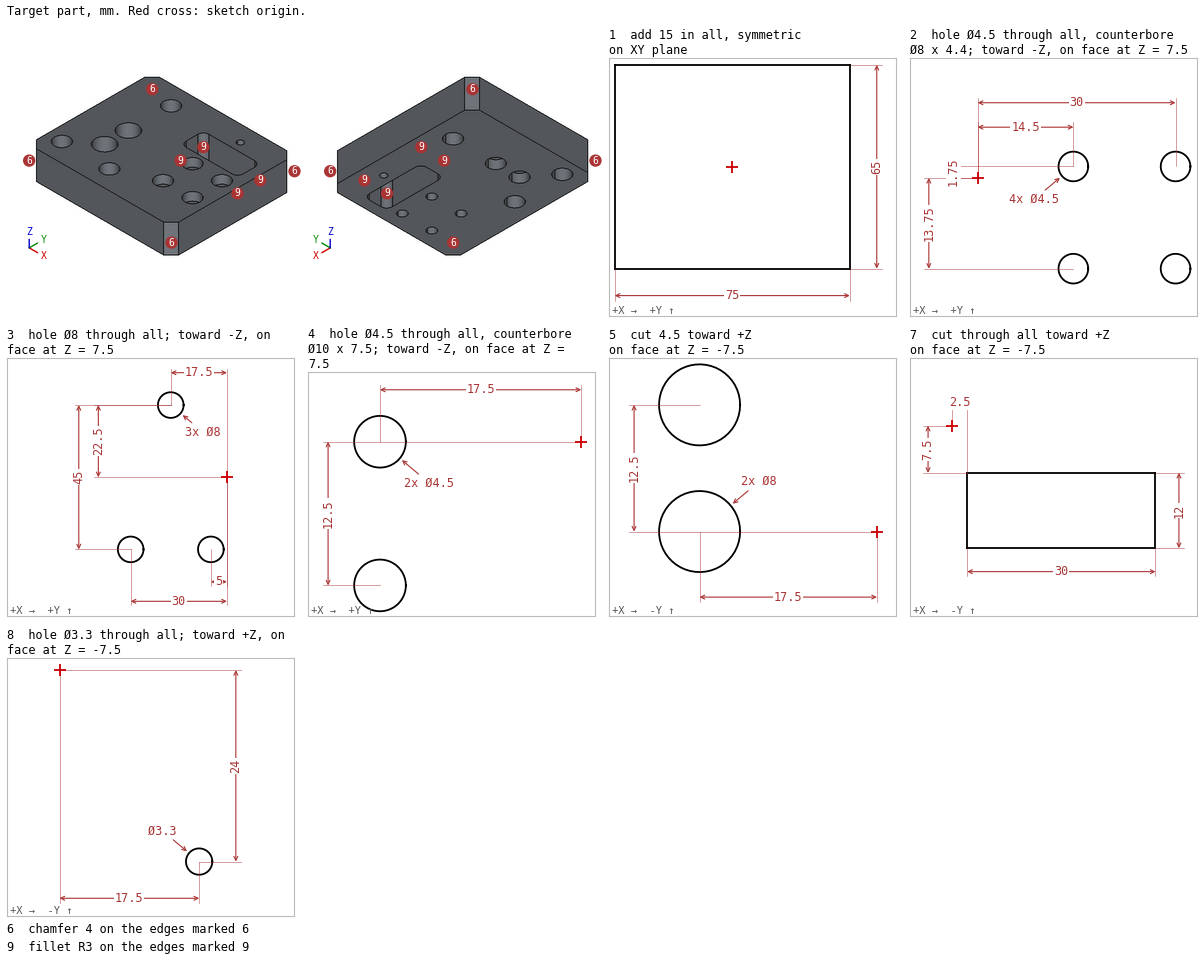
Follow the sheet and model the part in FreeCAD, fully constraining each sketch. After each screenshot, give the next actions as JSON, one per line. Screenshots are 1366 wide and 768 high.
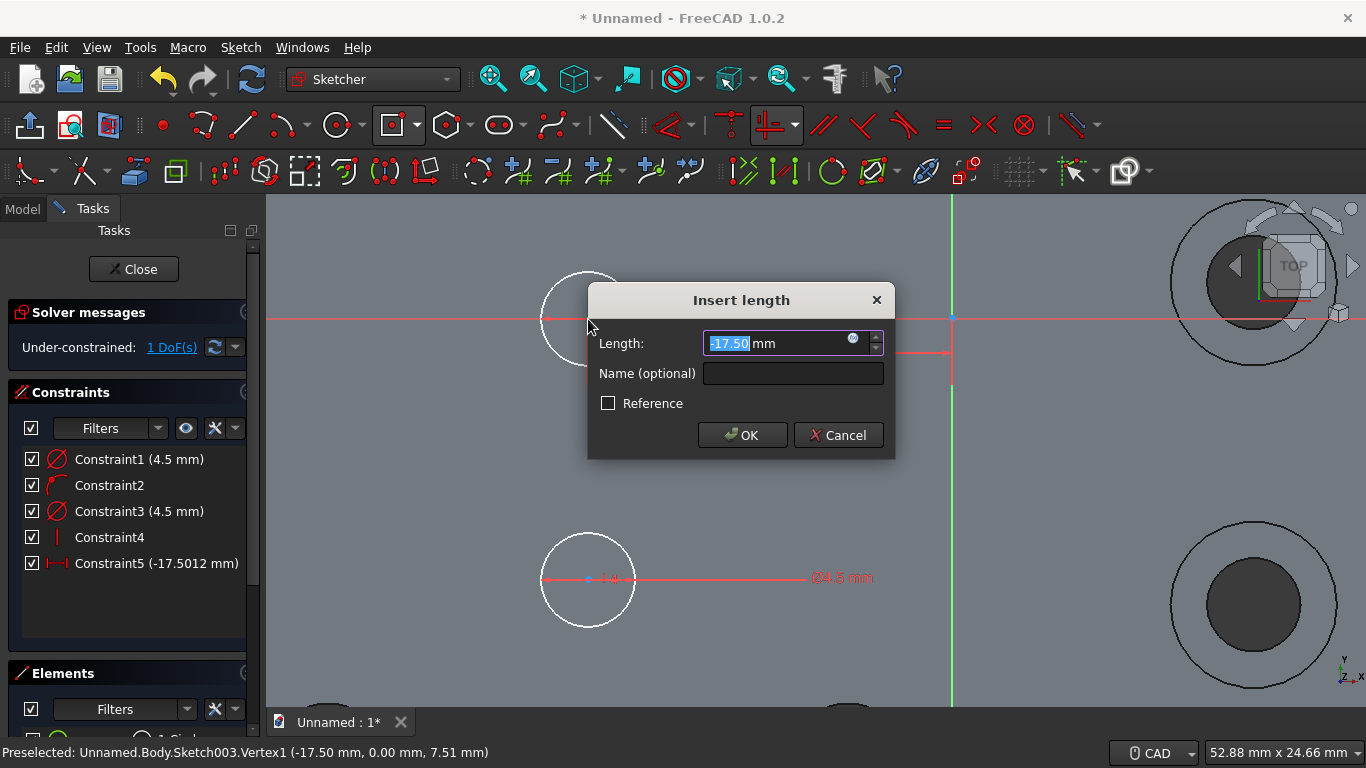
{"action": "type", "text": "-17.5"}
{"action": "key", "text": "Return"}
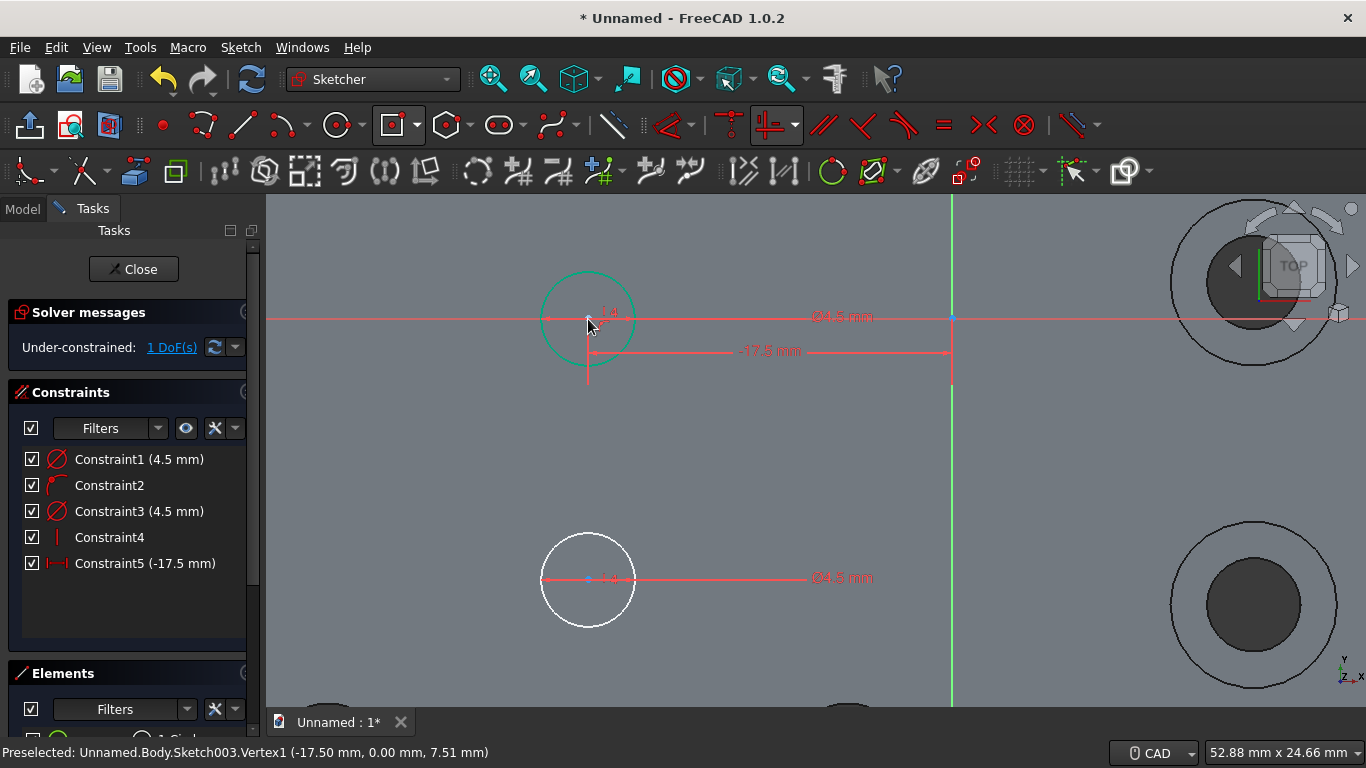
{"action": "left_click", "coordinate": [588, 580]}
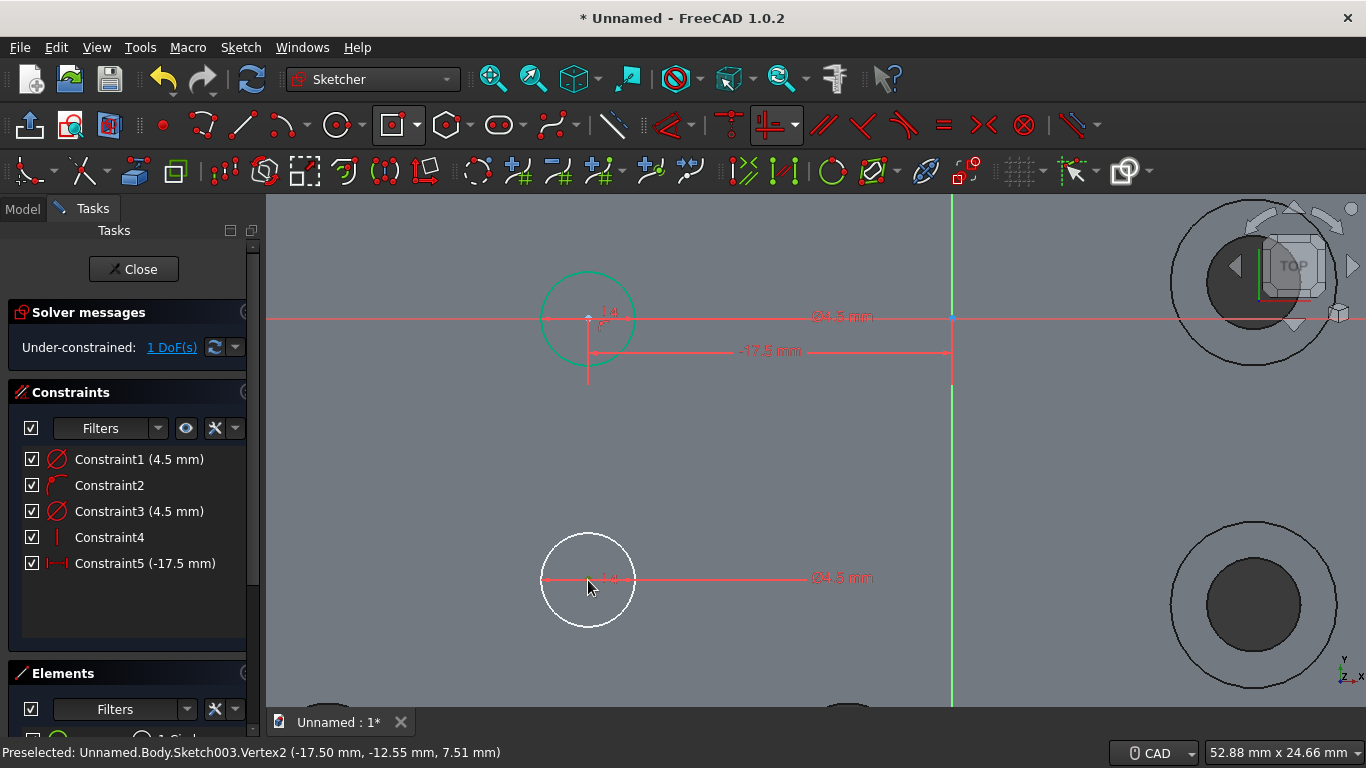
{"action": "key", "text": "i"}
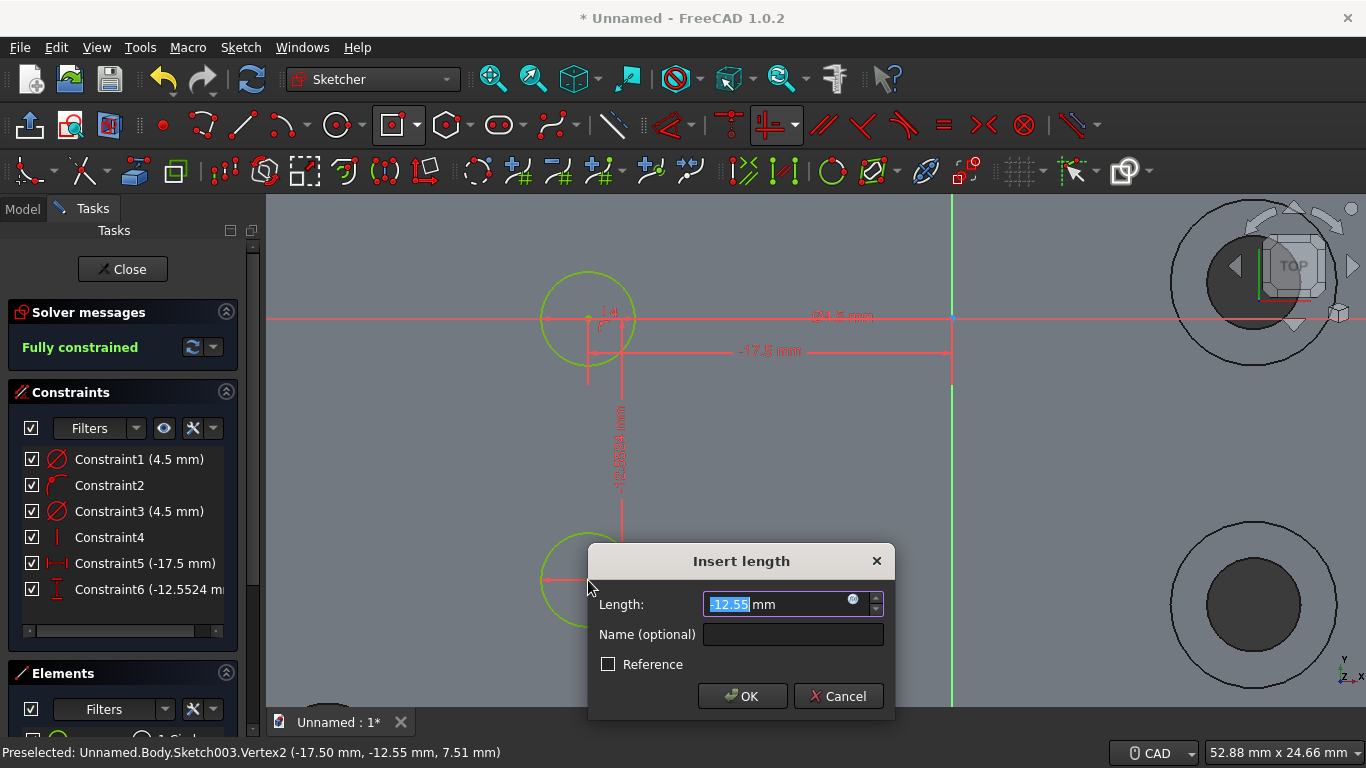
{"action": "type", "text": "-12.5"}
{"action": "key", "text": "Return"}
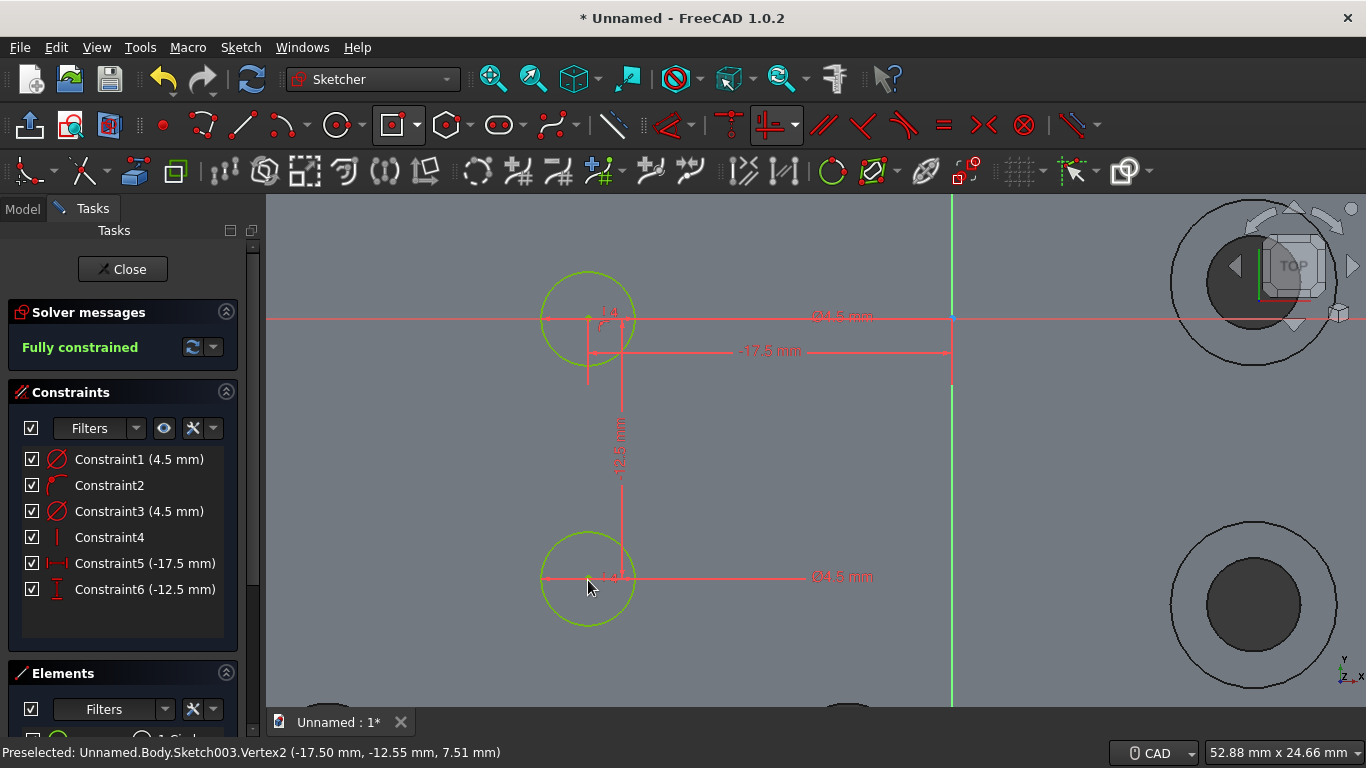
{"action": "left_click", "coordinate": [123, 269]}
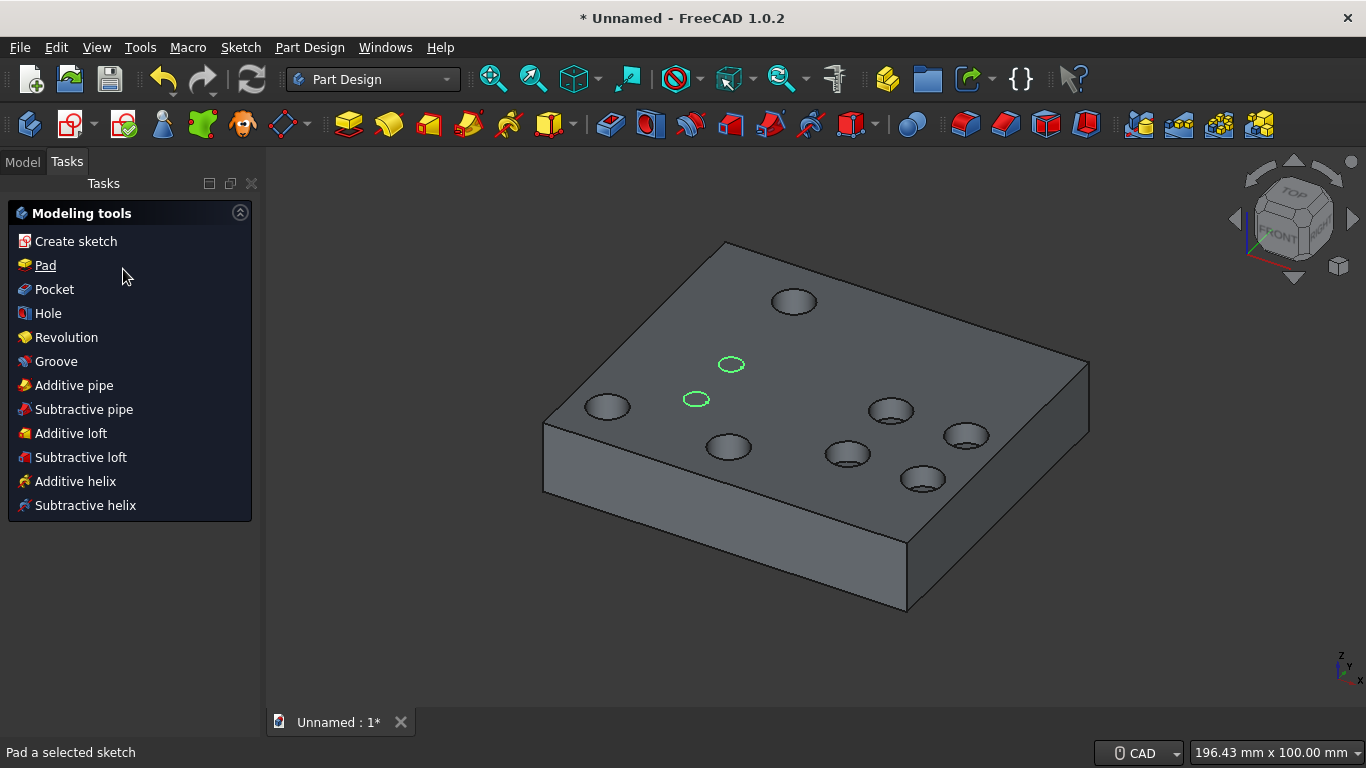
{"action": "left_click", "coordinate": [652, 124]}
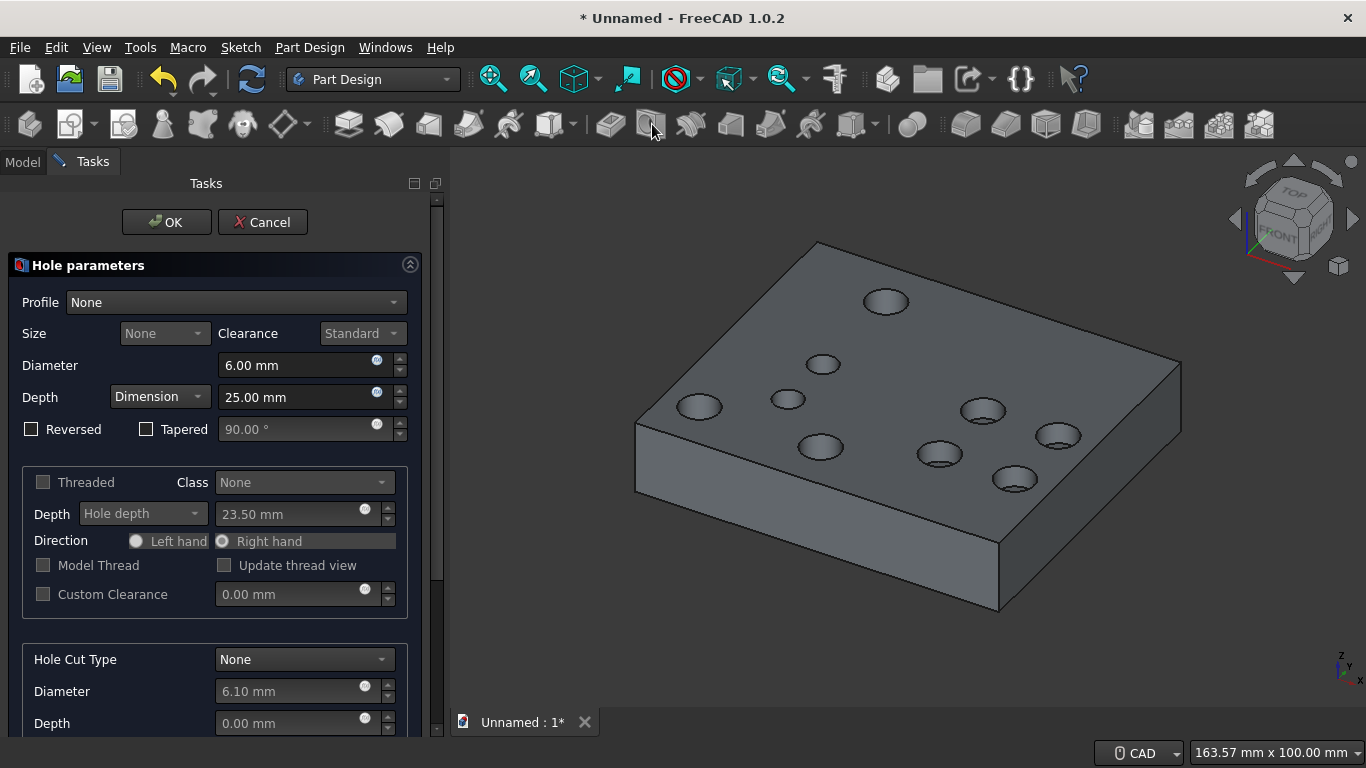
{"action": "triple_click", "coordinate": [305, 365]}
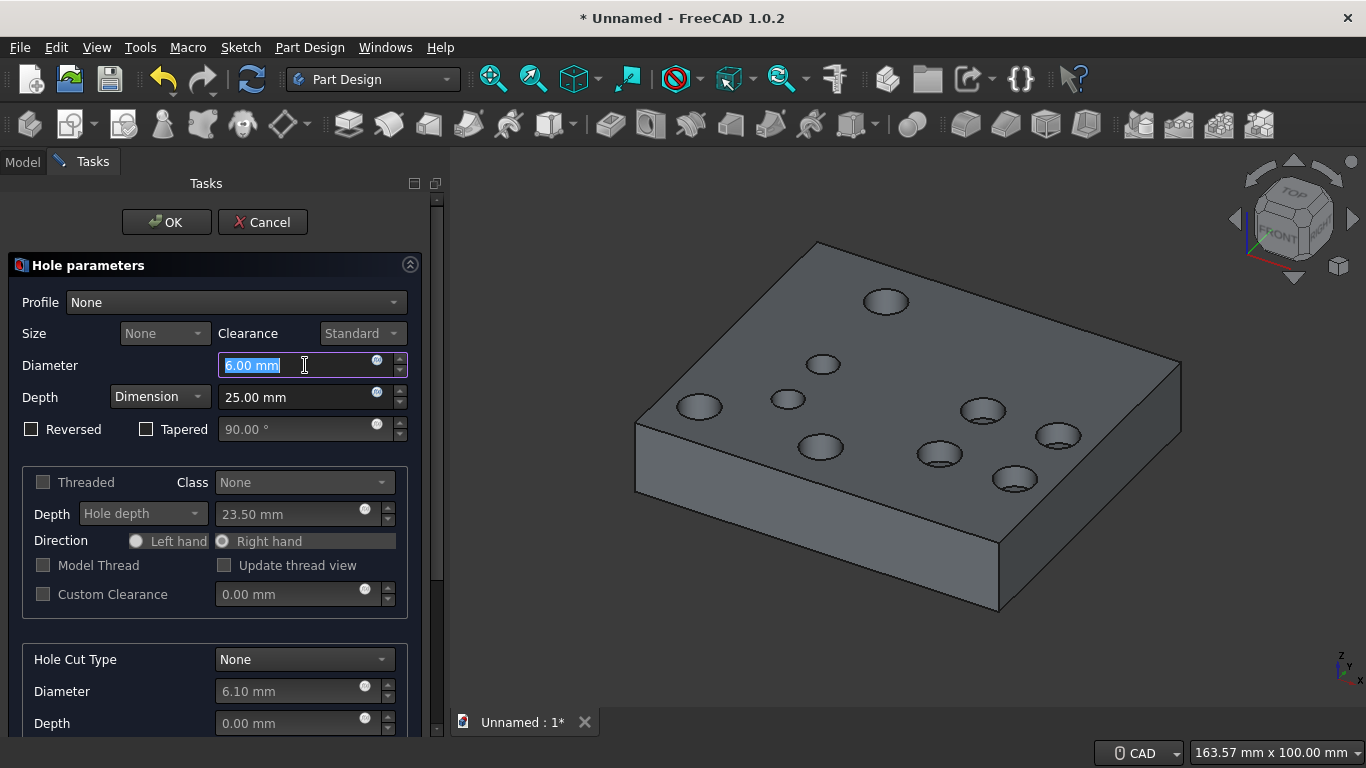
{"action": "type", "text": "4.5"}
{"action": "key", "text": "Tab"}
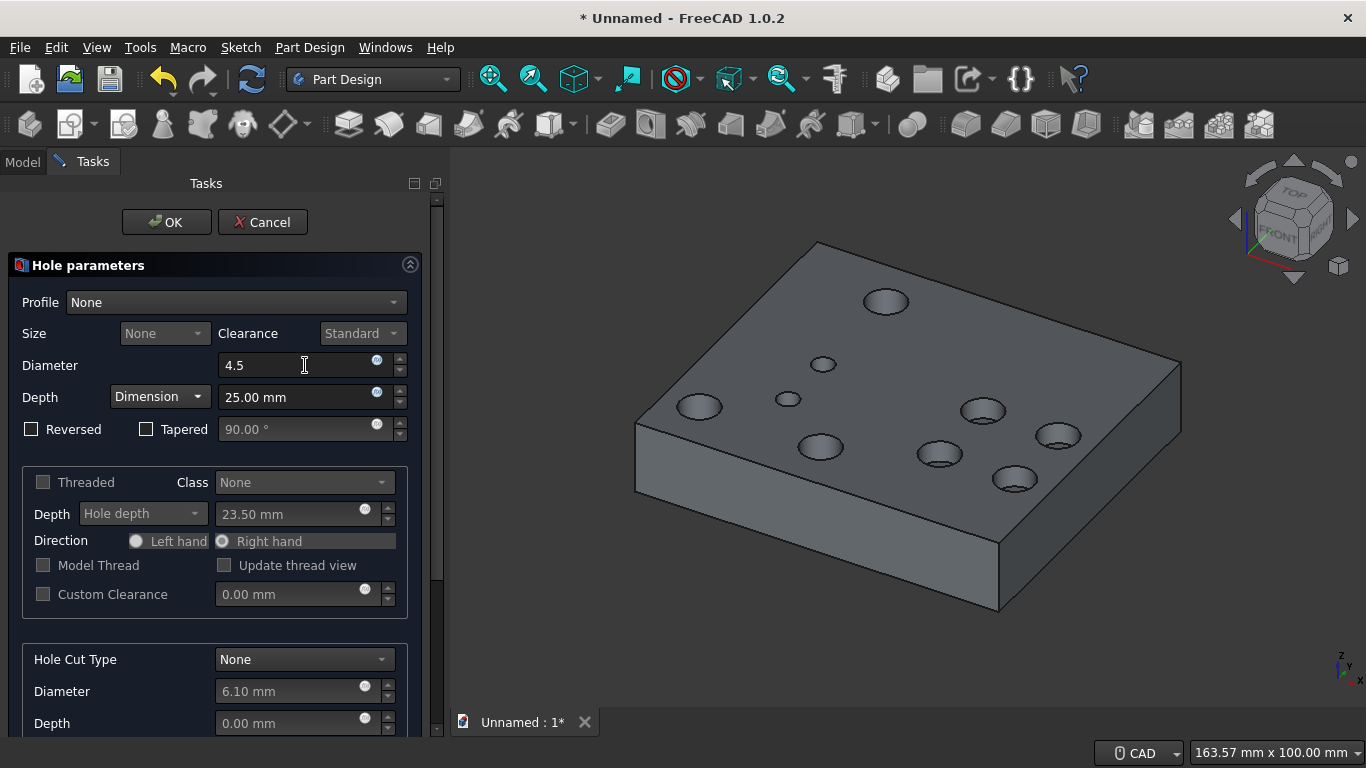
{"action": "left_click", "coordinate": [161, 396]}